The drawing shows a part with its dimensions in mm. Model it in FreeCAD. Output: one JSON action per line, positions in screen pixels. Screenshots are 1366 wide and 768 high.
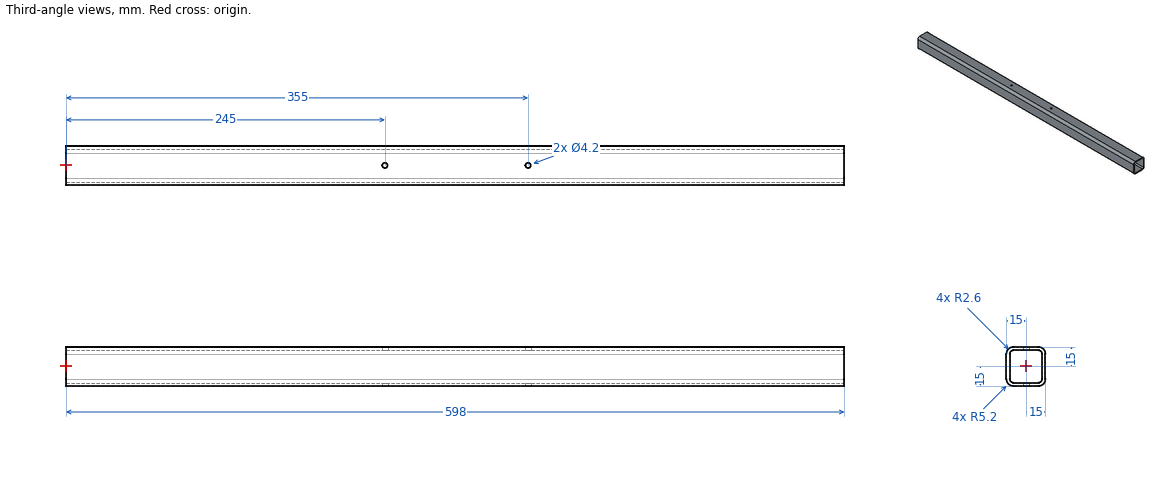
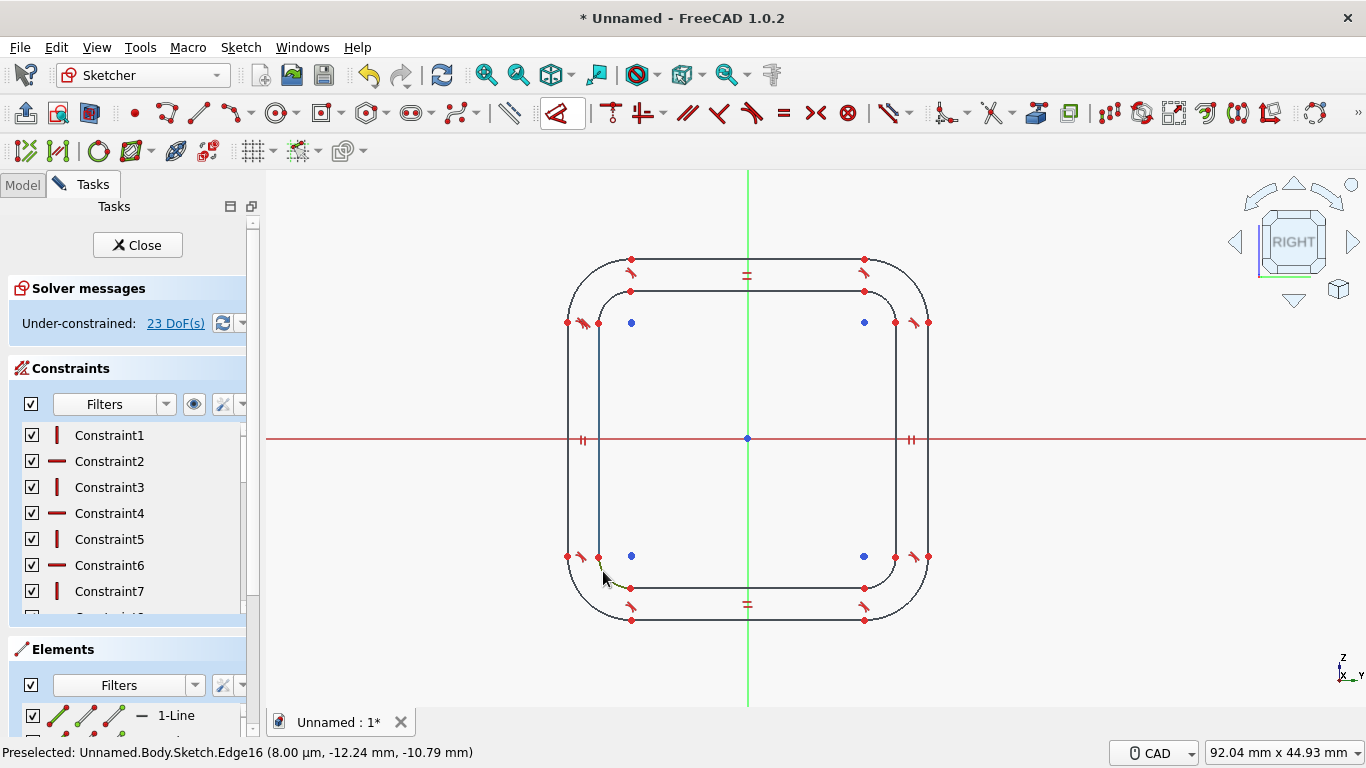
{"action": "left_click", "coordinate": [752, 114]}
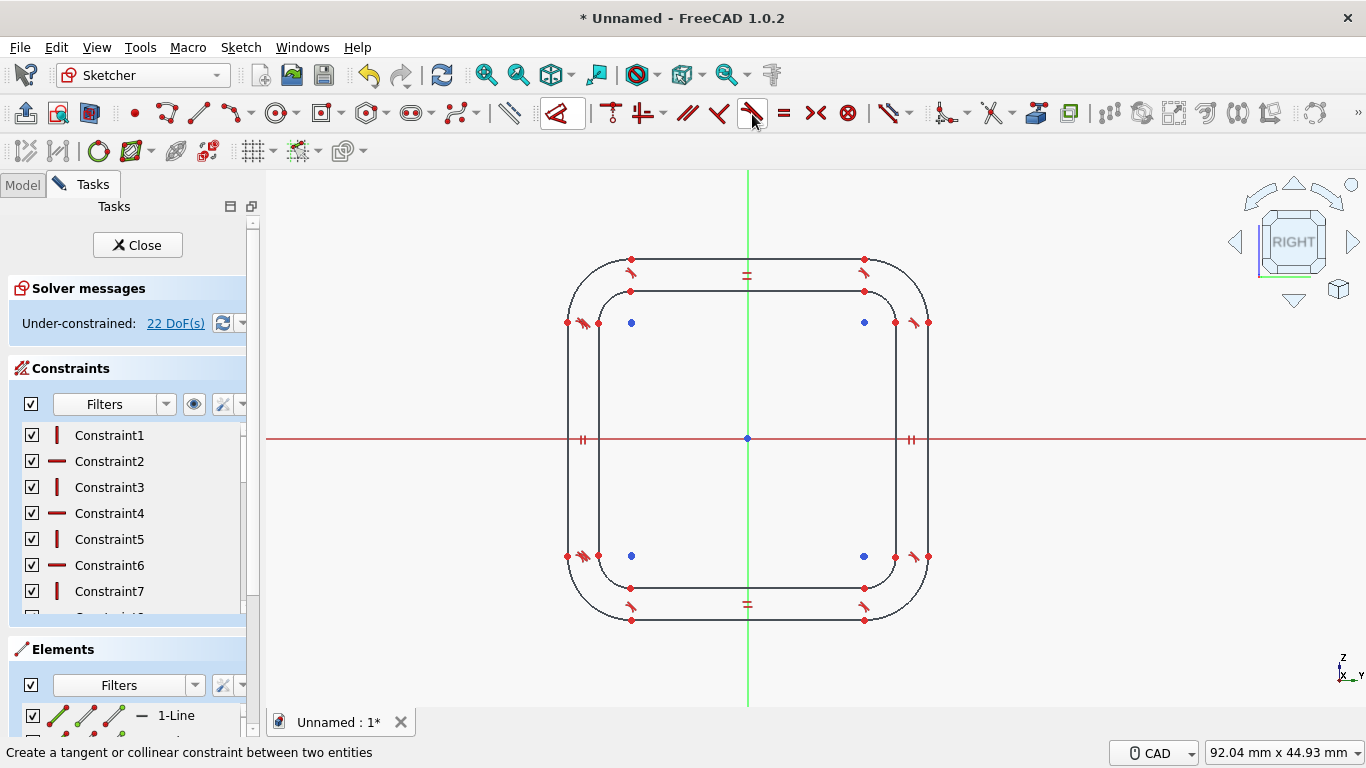
{"action": "left_click", "coordinate": [701, 291]}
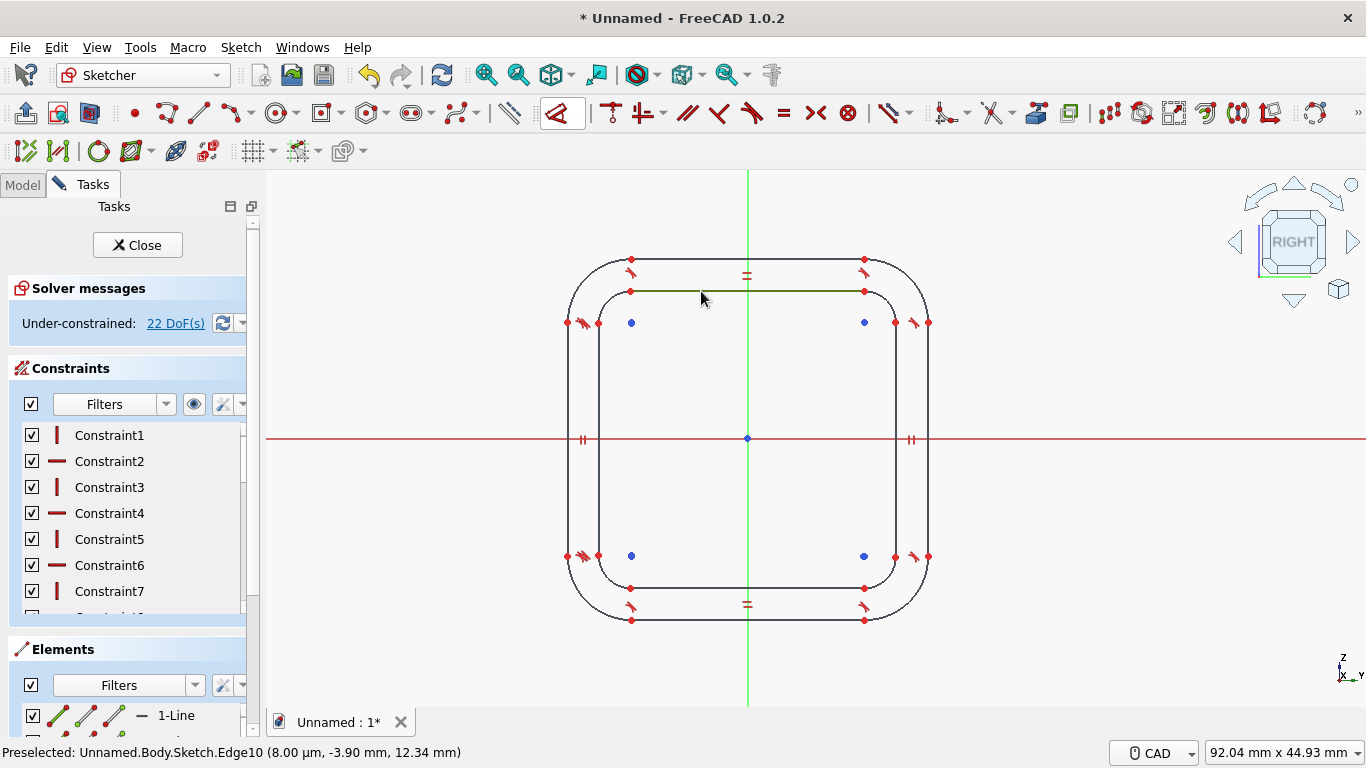
{"action": "left_click", "coordinate": [616, 295]}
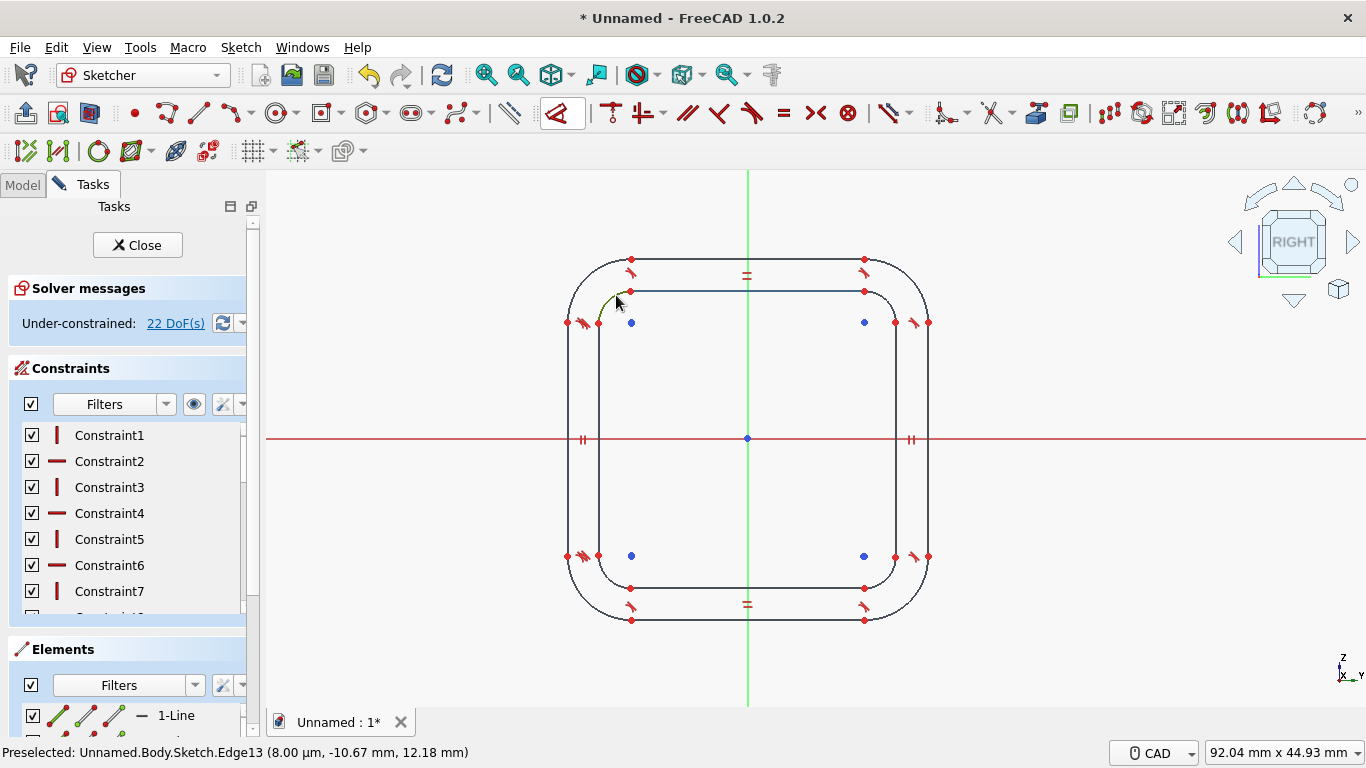
{"action": "key", "text": "t"}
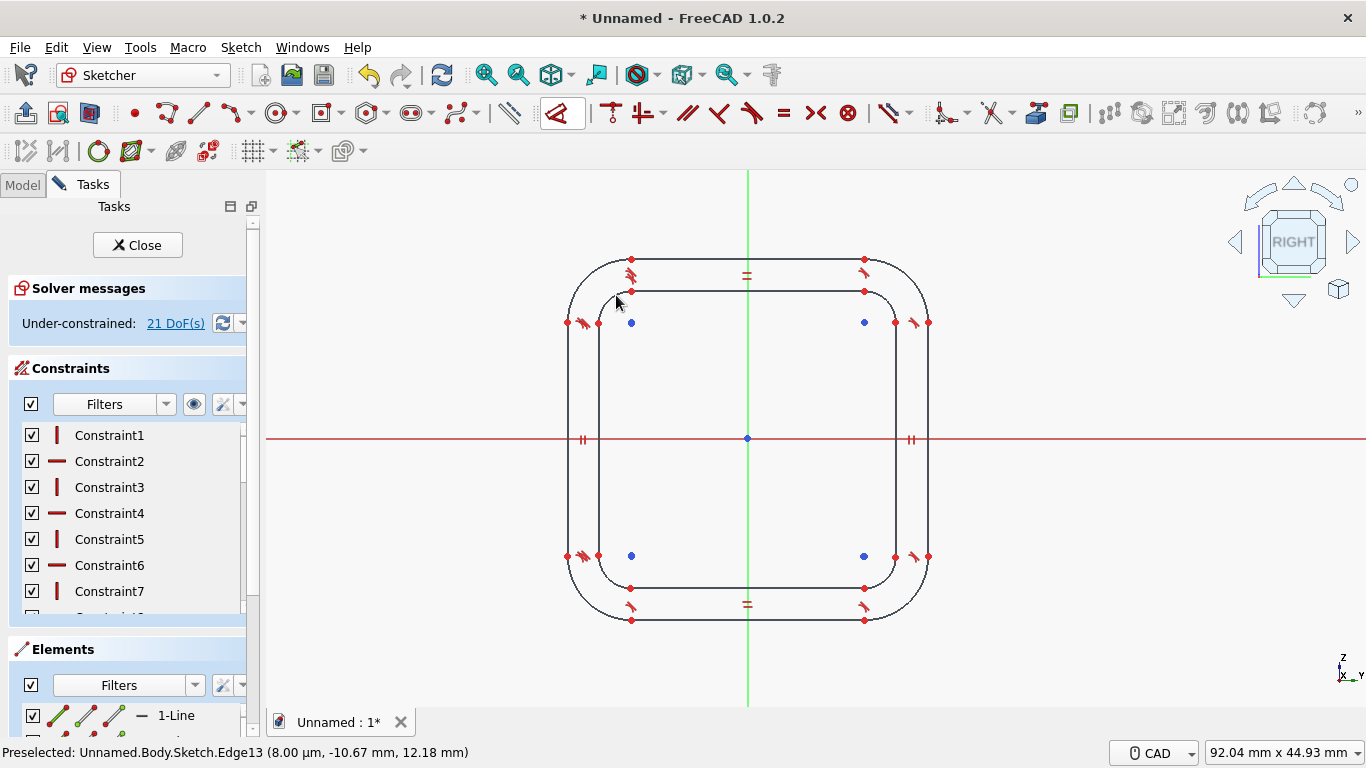
{"action": "left_click", "coordinate": [701, 291]}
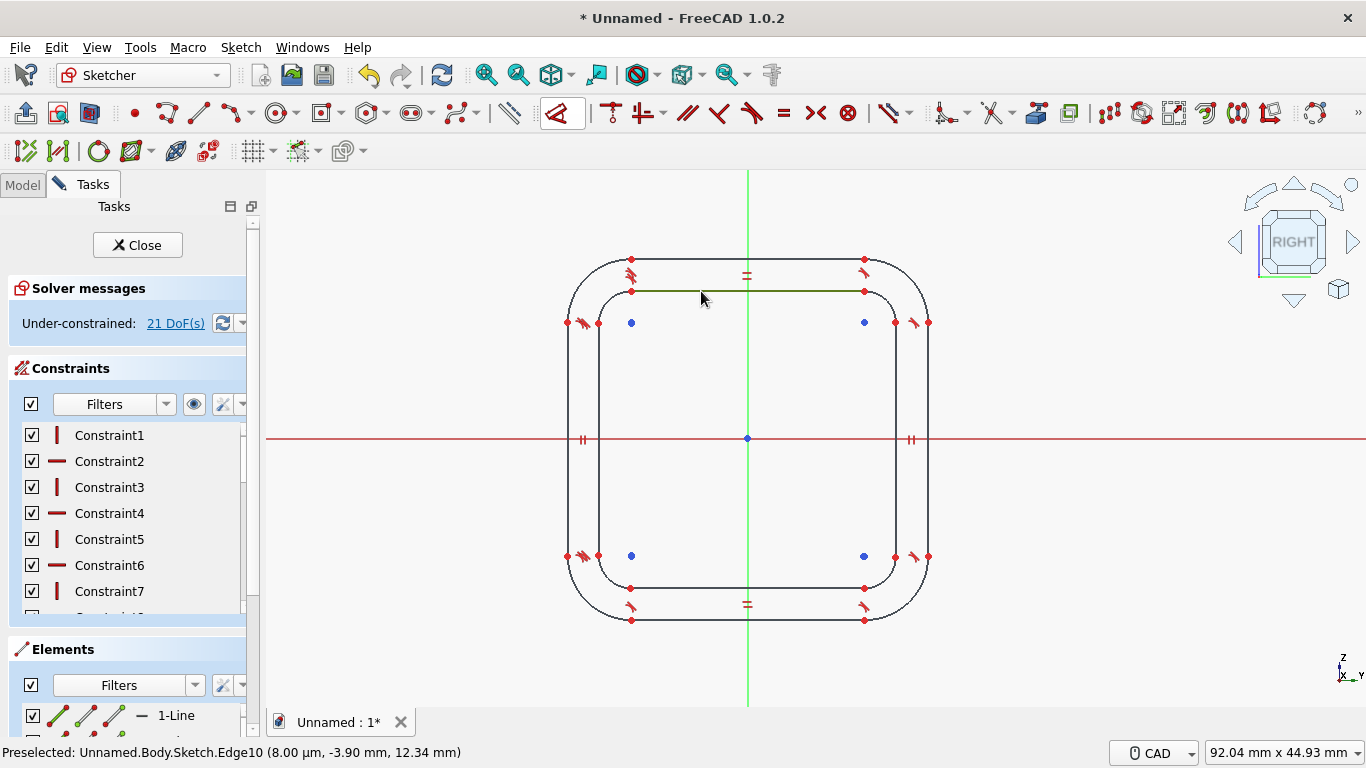
{"action": "left_click", "coordinate": [892, 308]}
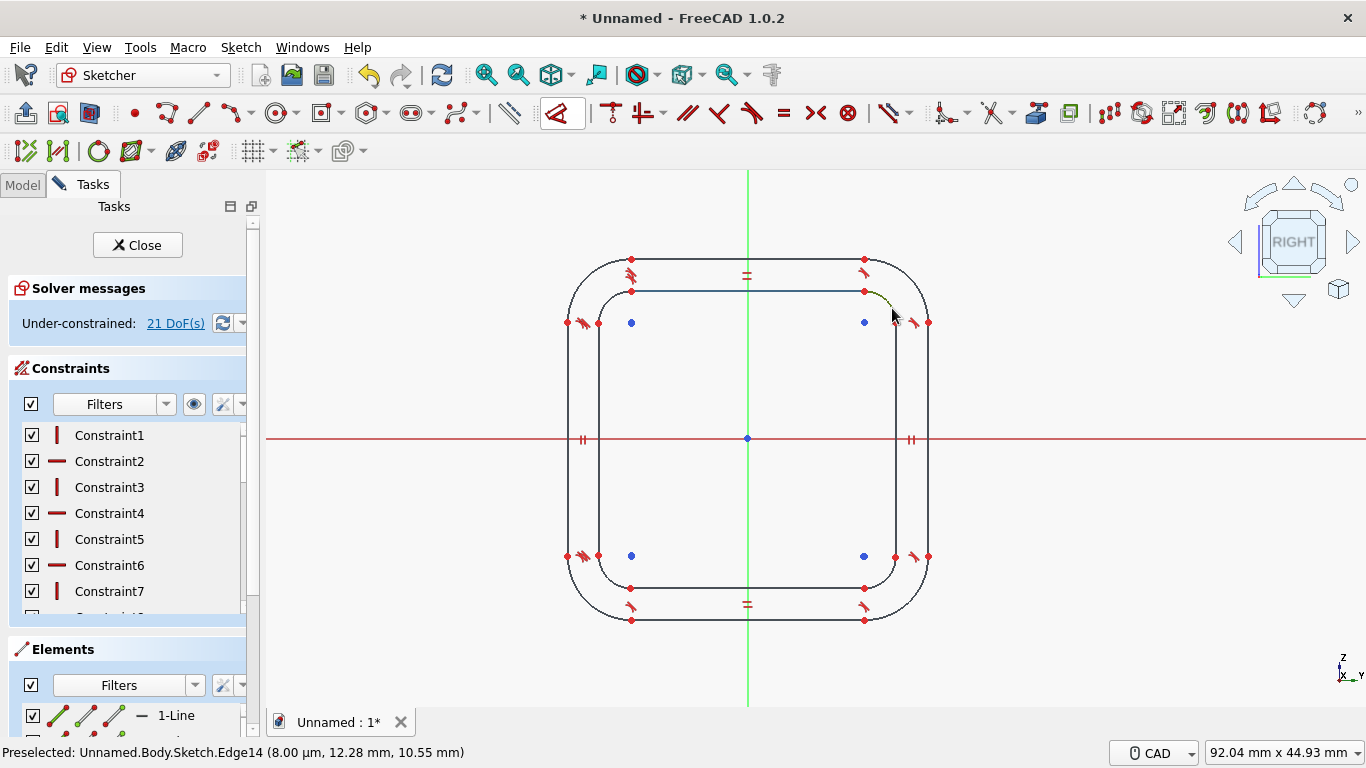
{"action": "left_click", "coordinate": [752, 114]}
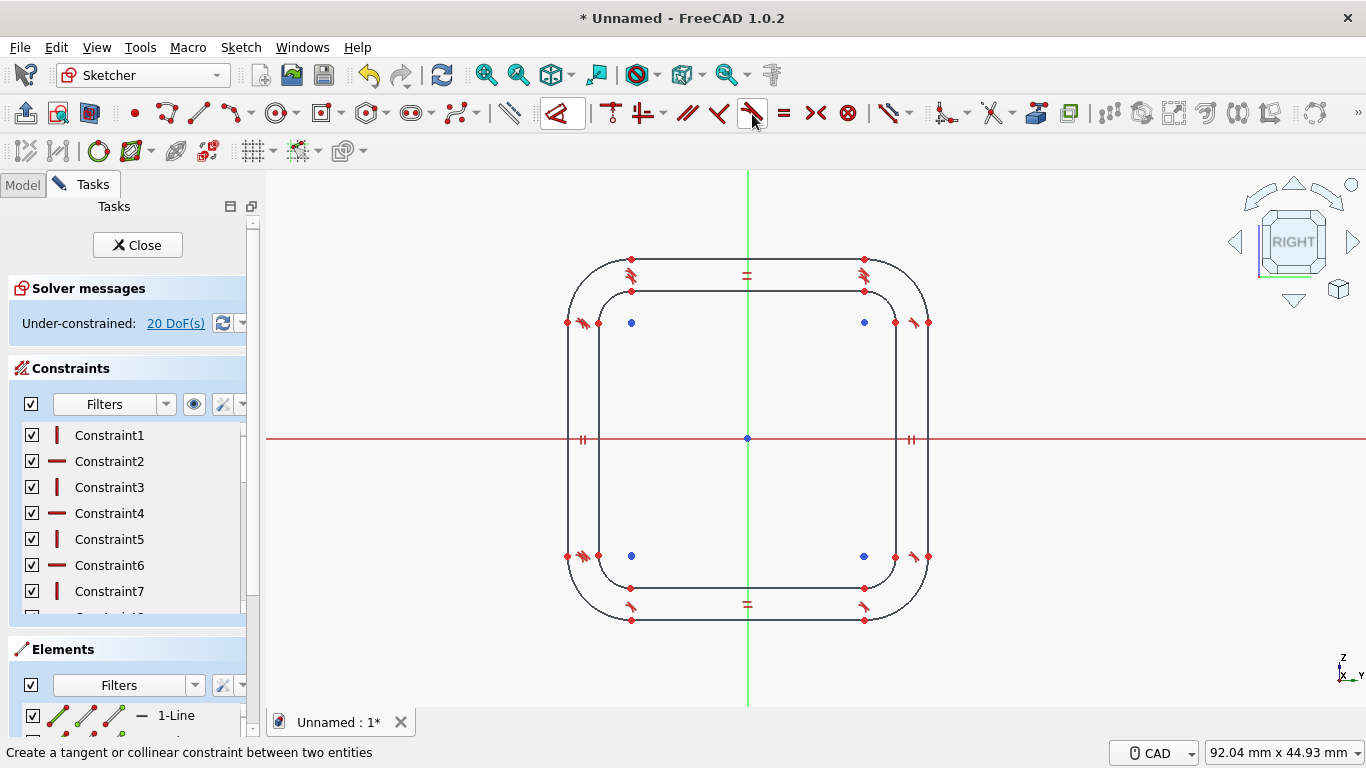
{"action": "left_click", "coordinate": [896, 393]}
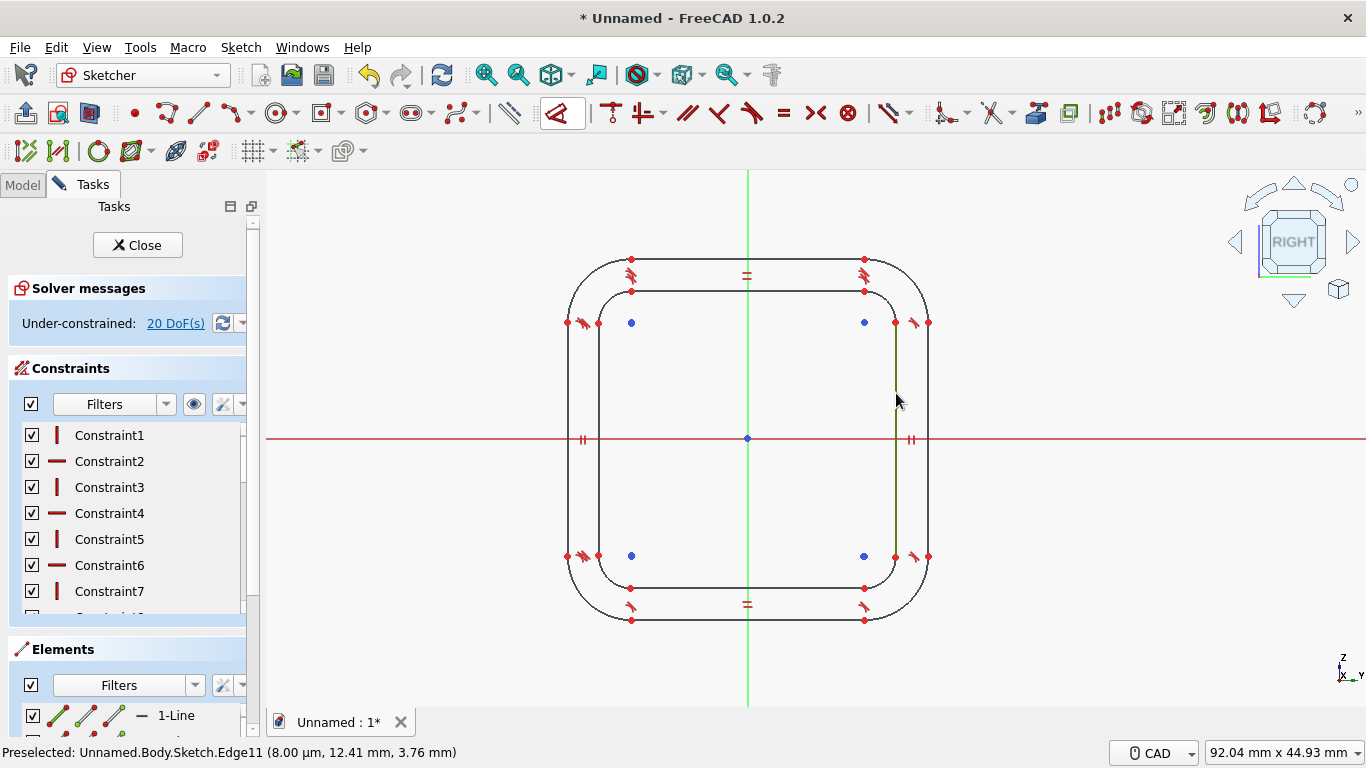
{"action": "left_click", "coordinate": [892, 308]}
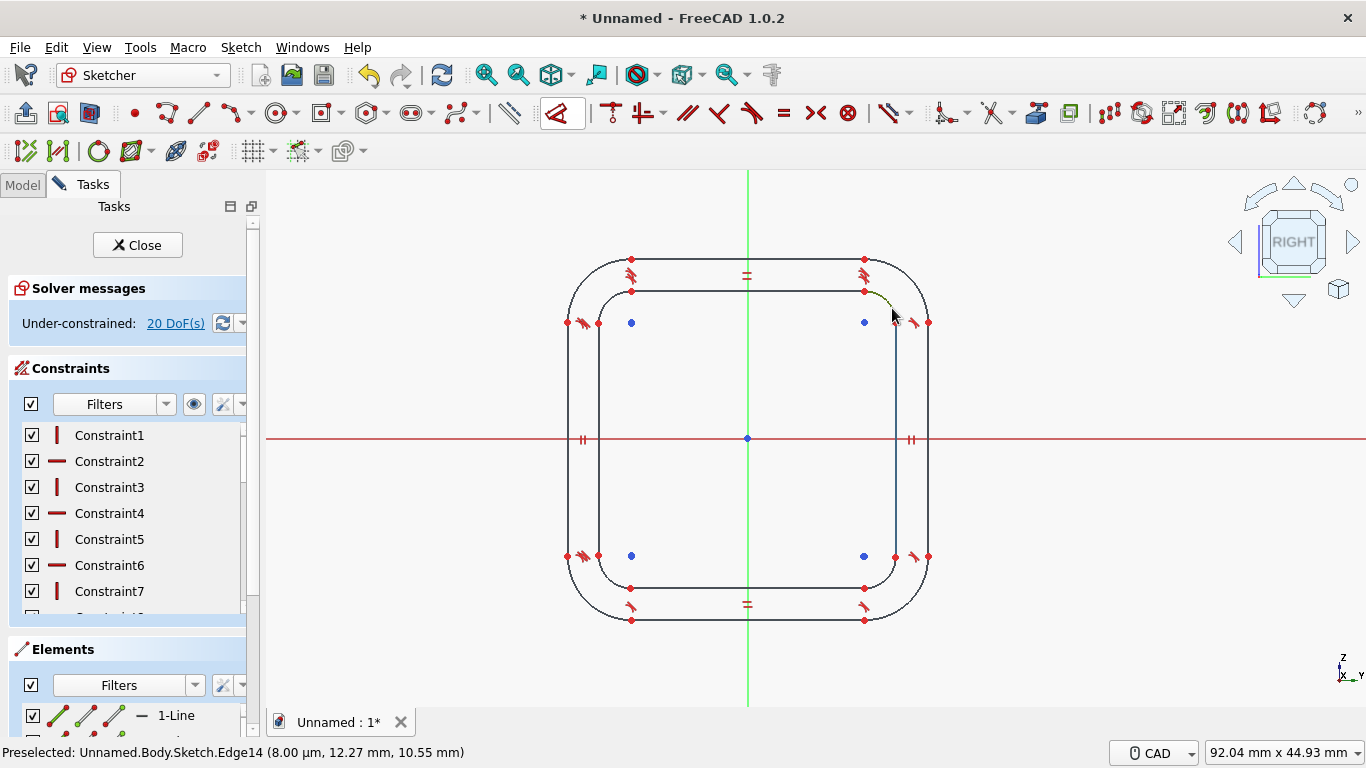
{"action": "key", "text": "t"}